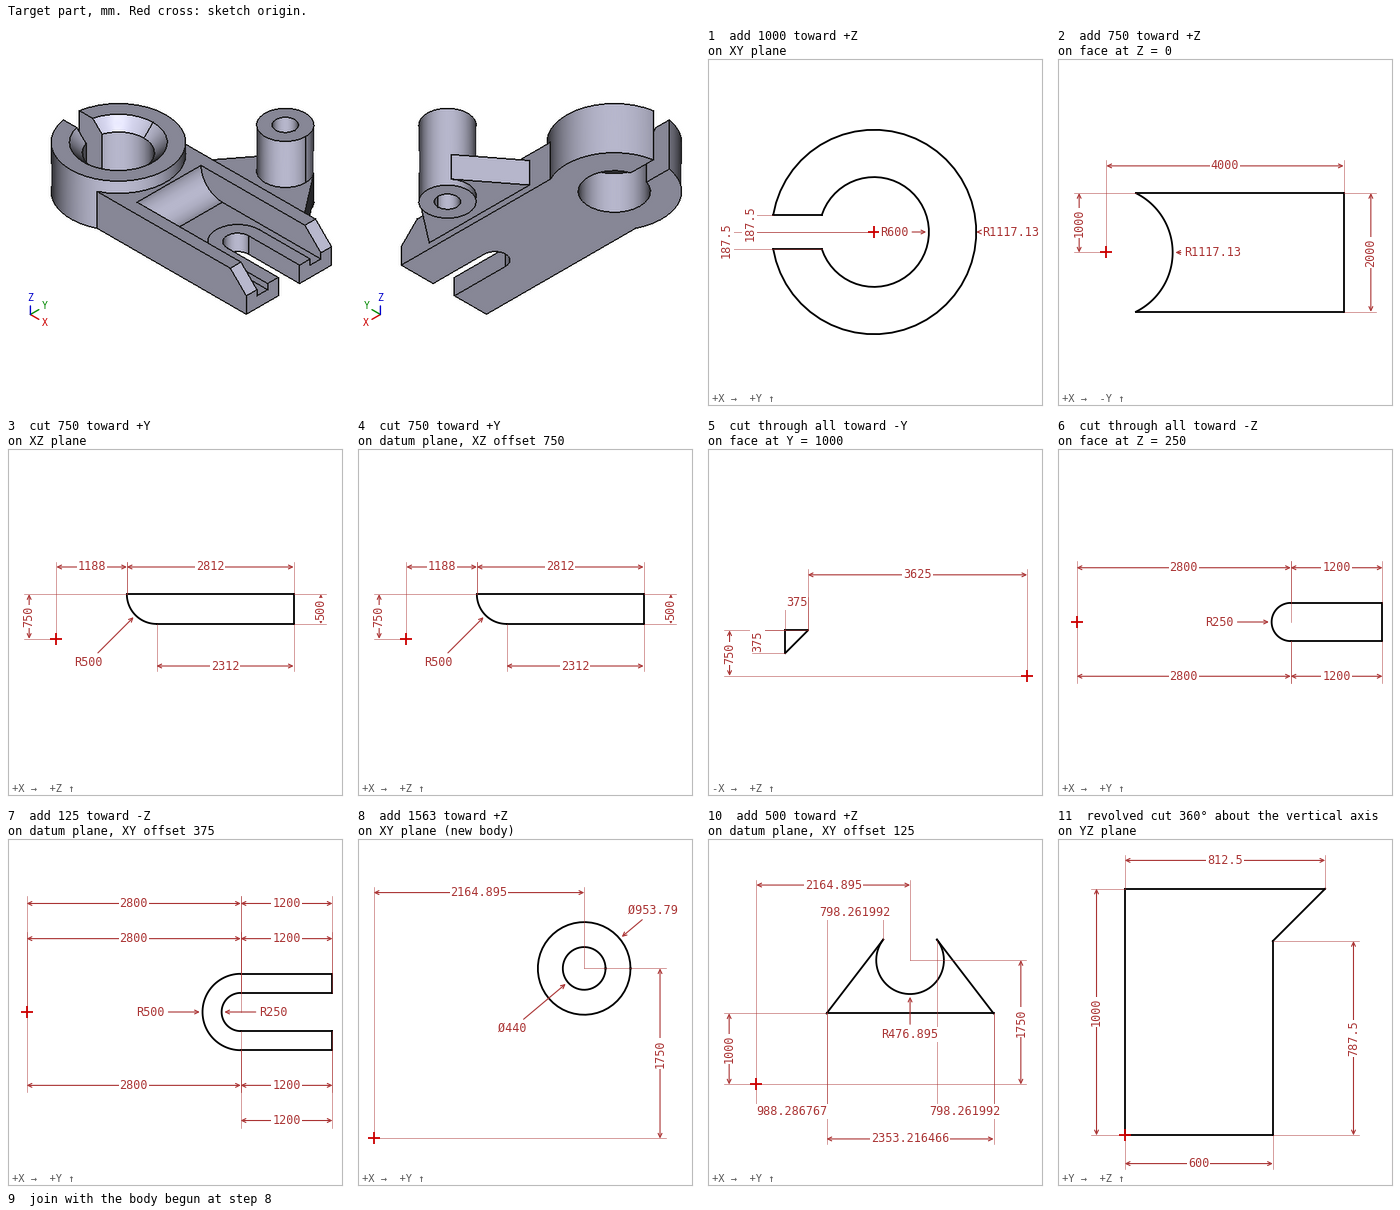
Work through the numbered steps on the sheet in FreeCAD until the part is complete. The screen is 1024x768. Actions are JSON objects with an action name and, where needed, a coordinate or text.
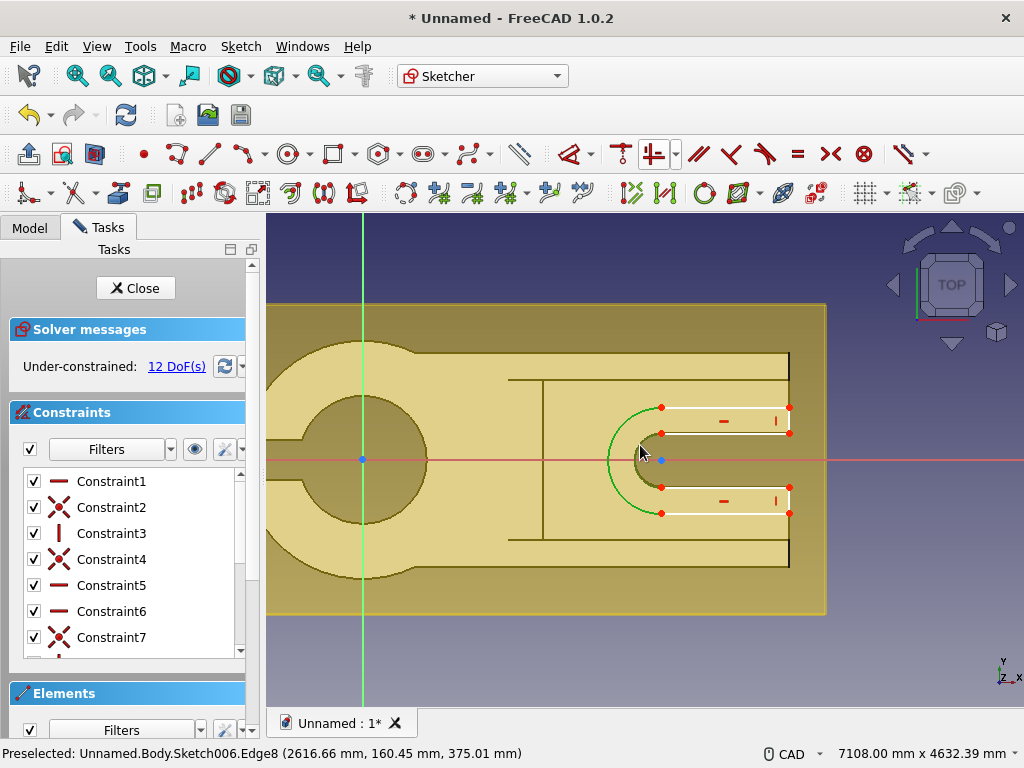
{"action": "key", "text": "c"}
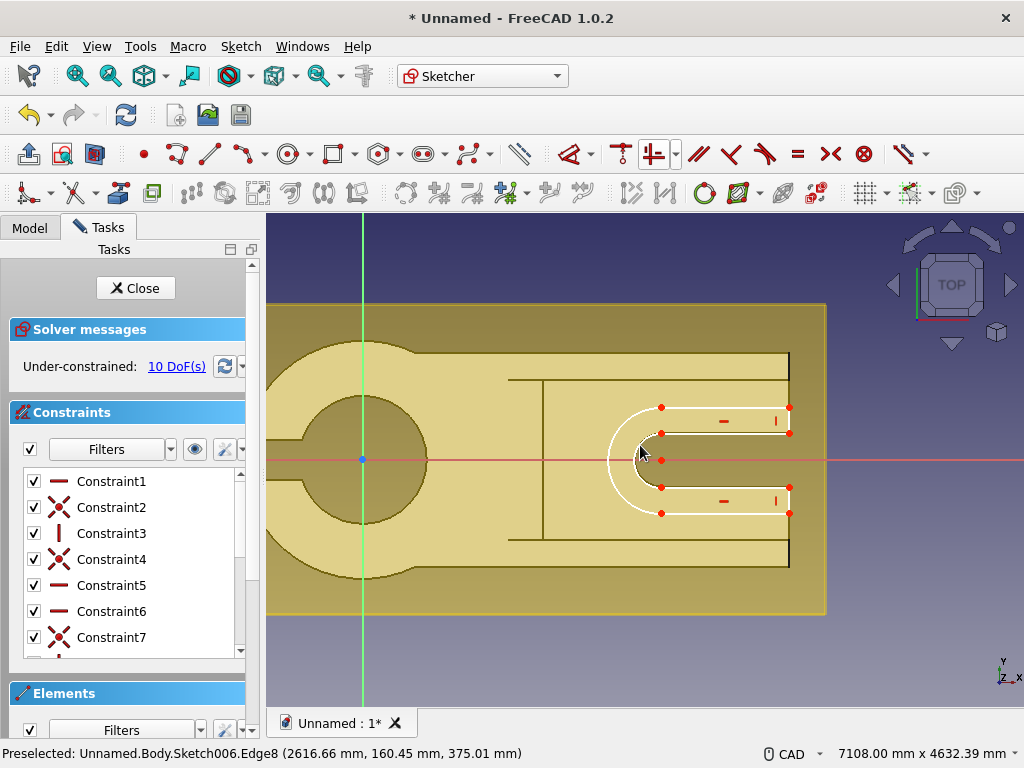
{"action": "left_click", "coordinate": [661, 461]}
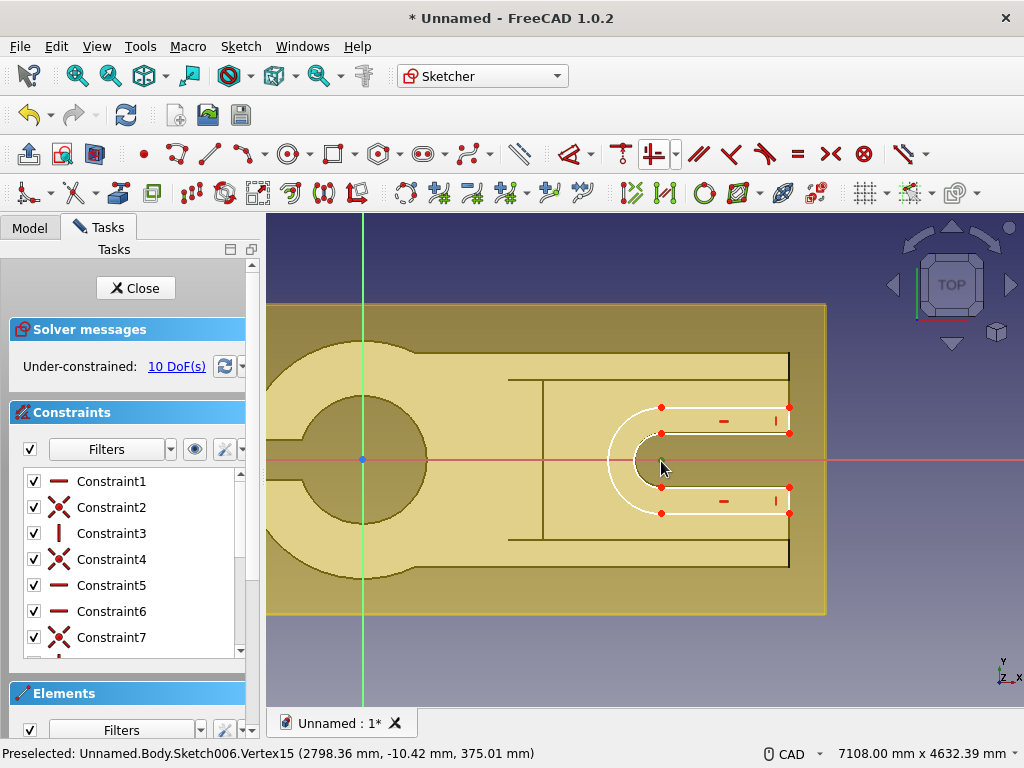
{"action": "left_click", "coordinate": [415, 460]}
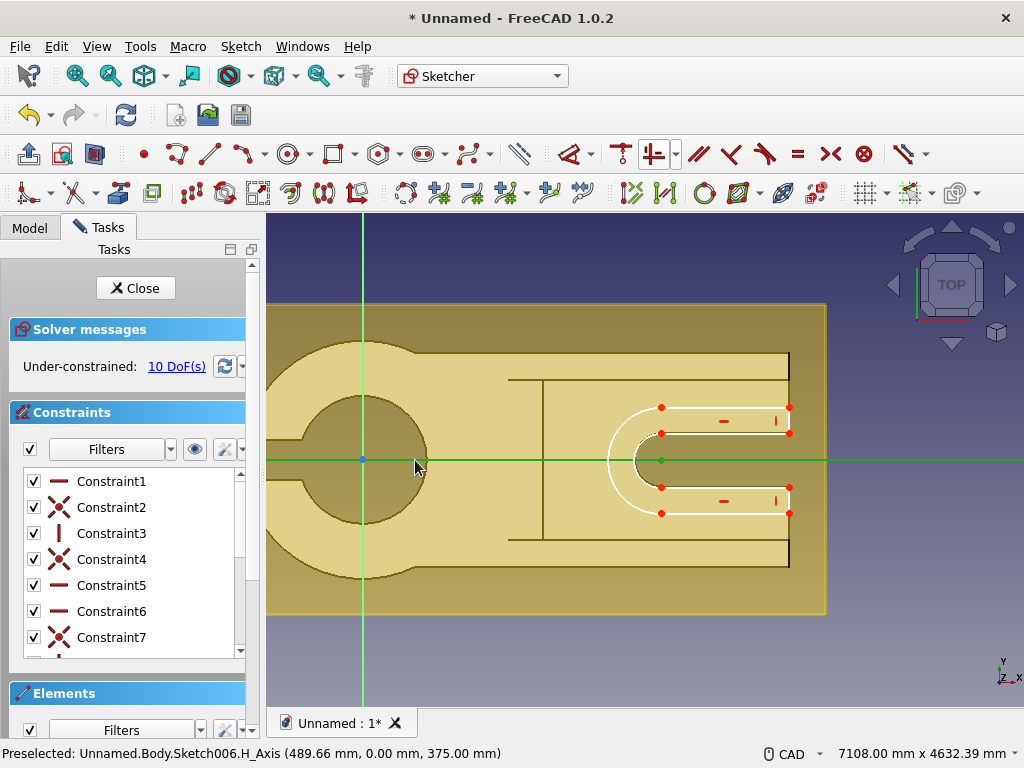
{"action": "key", "text": "c"}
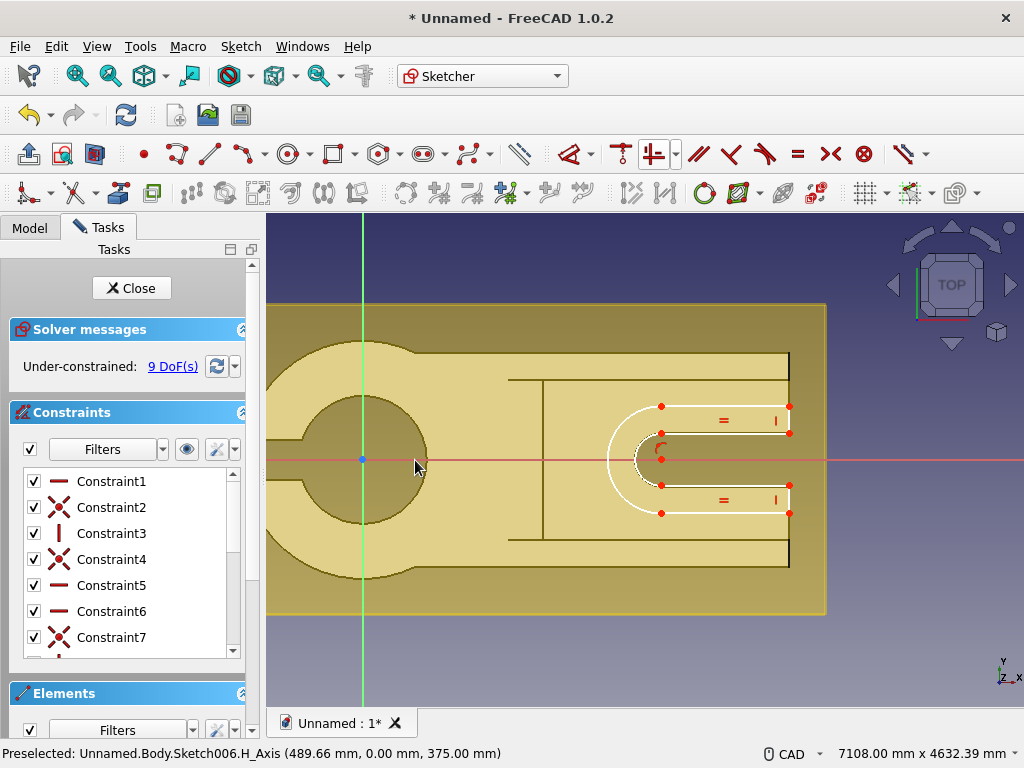
{"action": "key", "text": "d"}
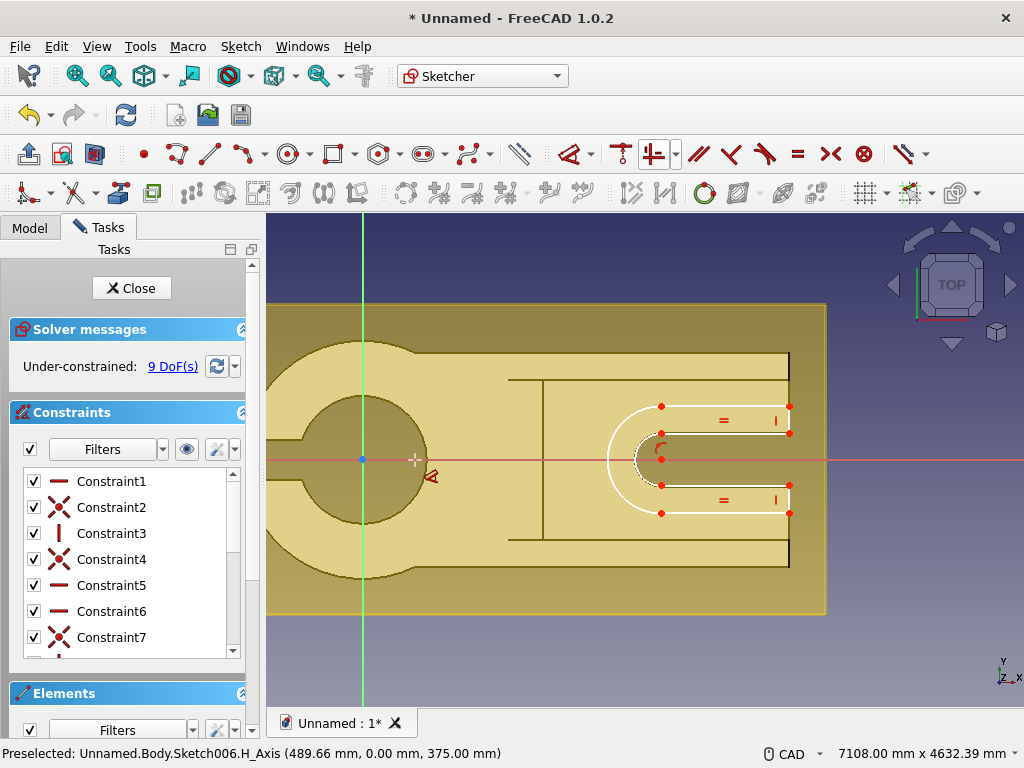
{"action": "left_click", "coordinate": [618, 428]}
{"action": "left_click", "coordinate": [592, 409]}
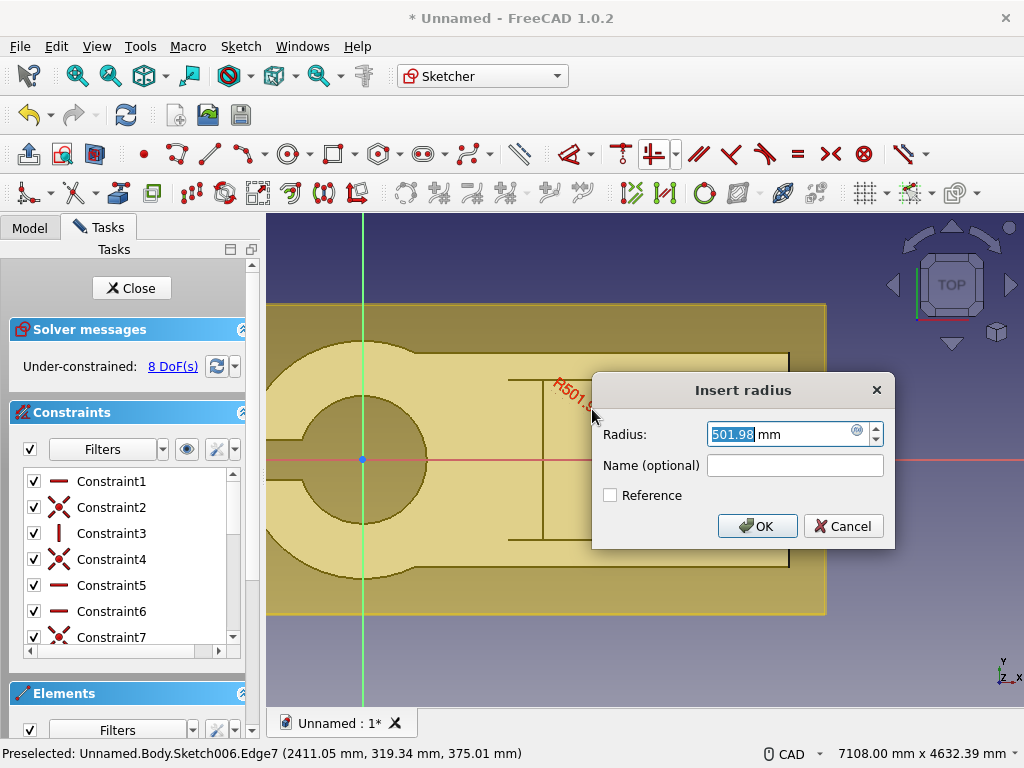
{"action": "type", "text": "500"}
{"action": "key", "text": "Return"}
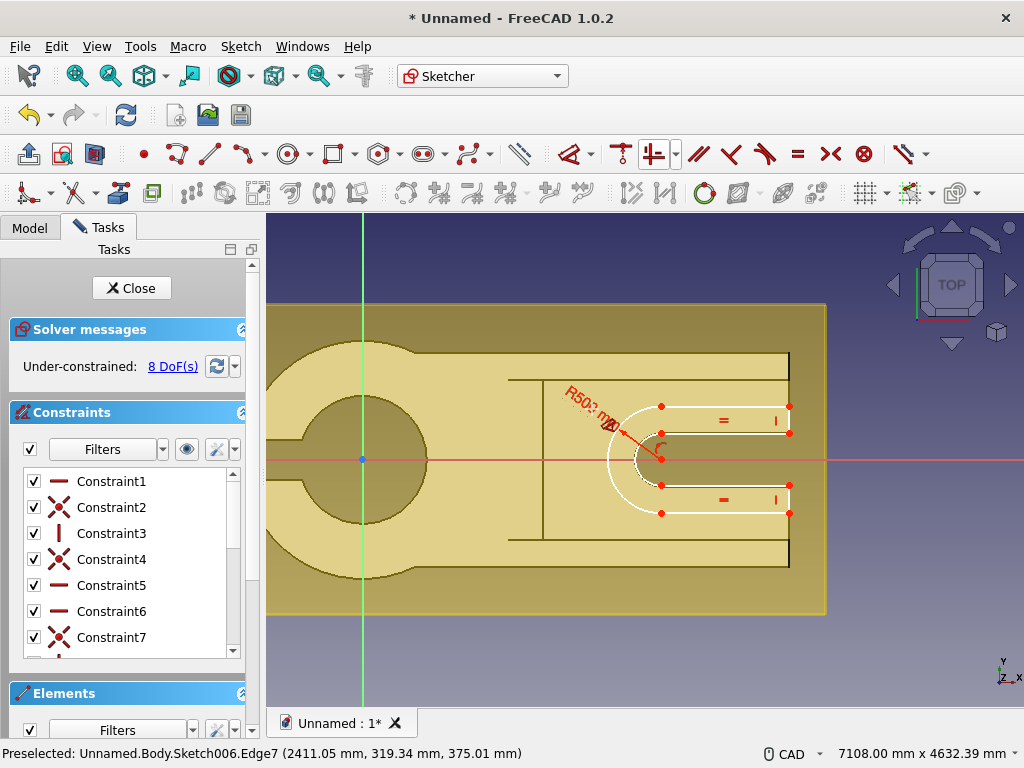
{"action": "scroll", "coordinate": [640, 445], "scroll_direction": "up", "scroll_amount": 2}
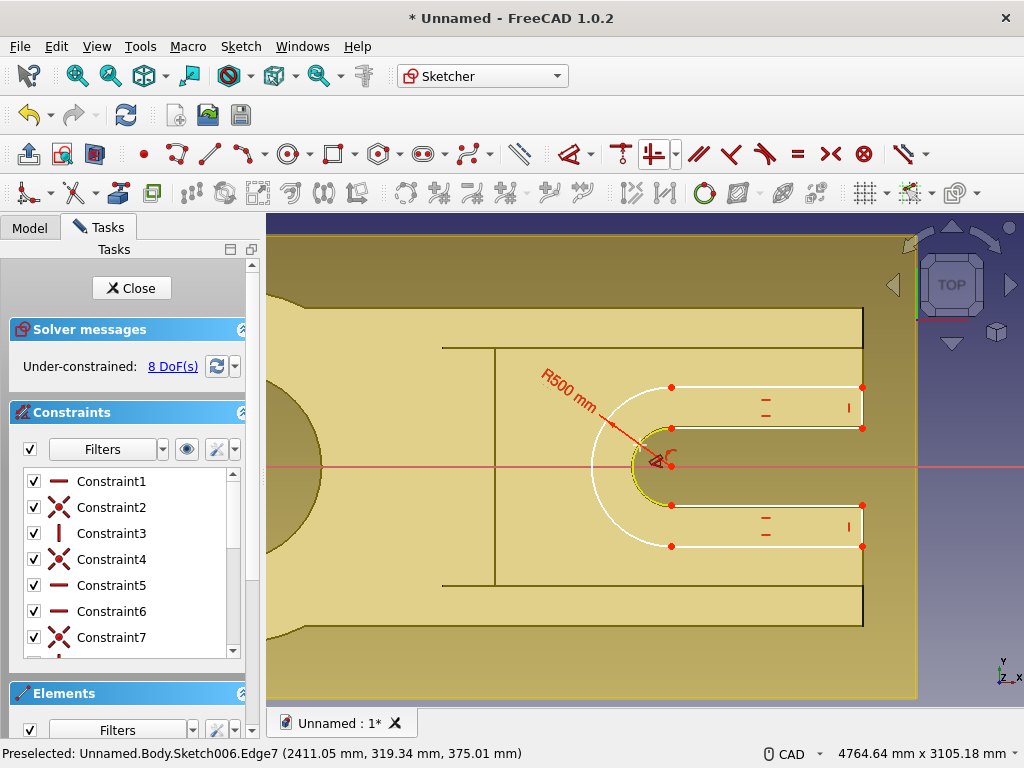
{"action": "left_click", "coordinate": [640, 444]}
{"action": "left_click", "coordinate": [713, 410]}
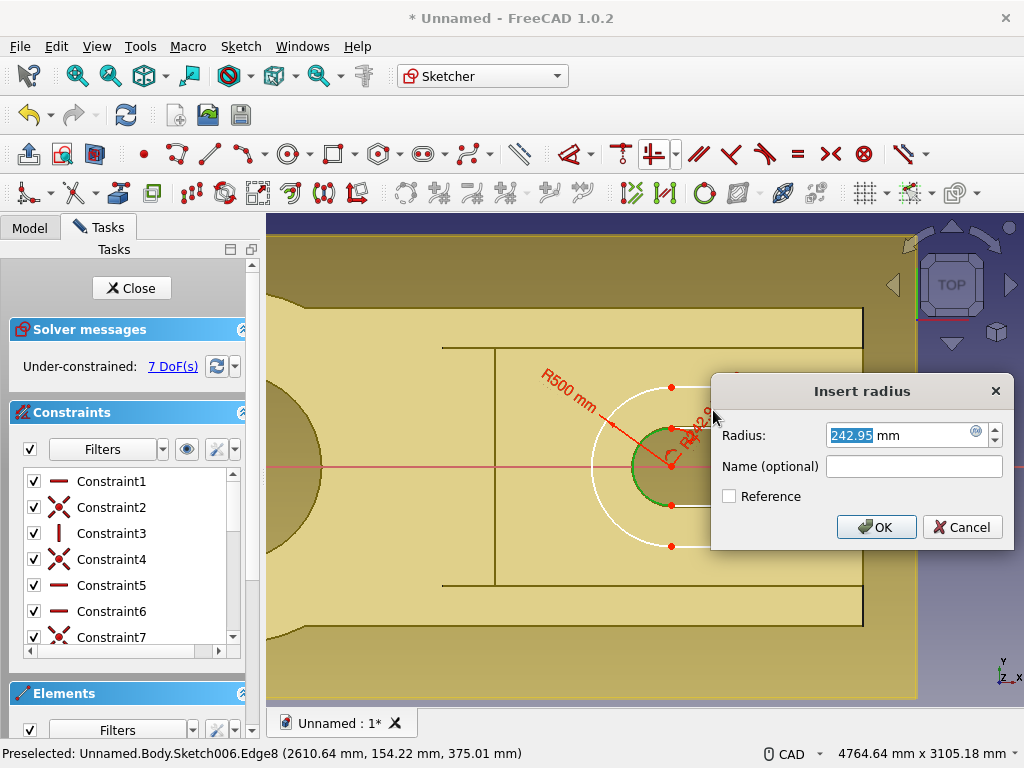
{"action": "type", "text": "250"}
{"action": "key", "text": "Return"}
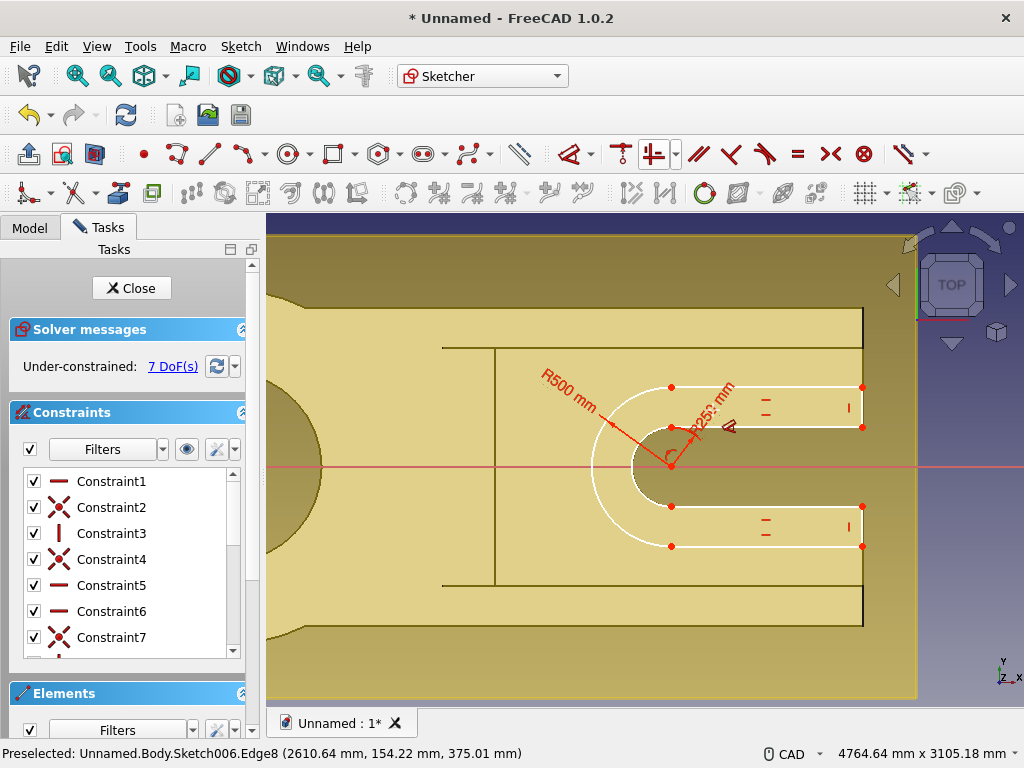
{"action": "left_click", "coordinate": [728, 427]}
{"action": "left_click", "coordinate": [765, 369]}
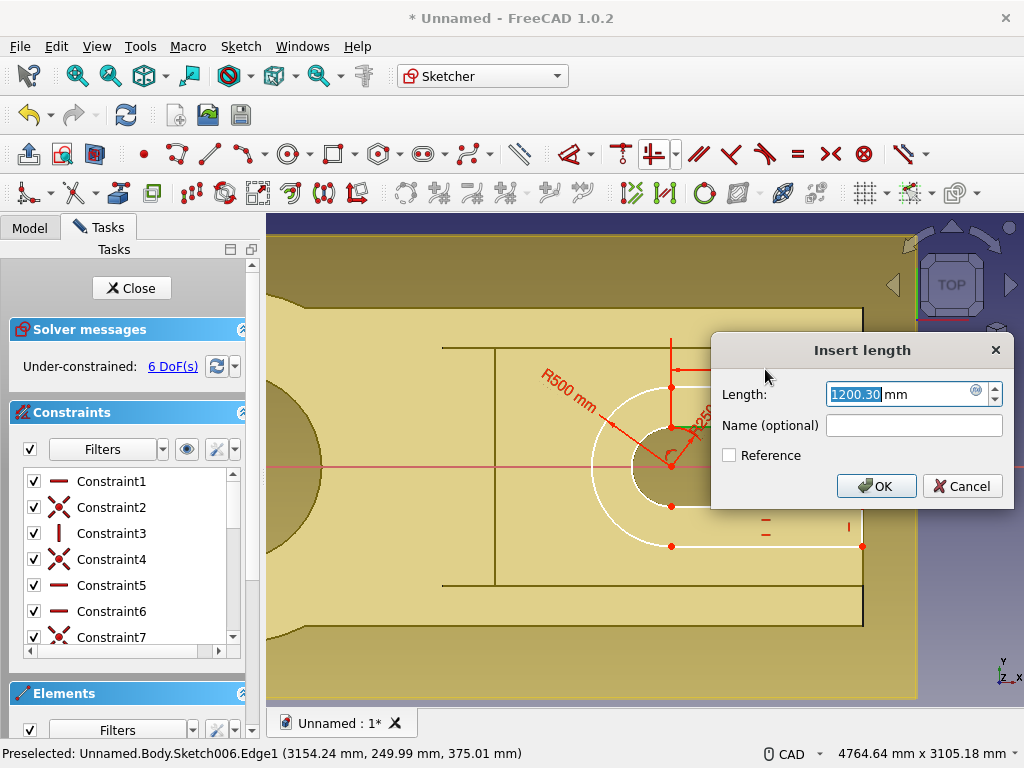
{"action": "type", "text": "1200"}
{"action": "key", "text": "Return"}